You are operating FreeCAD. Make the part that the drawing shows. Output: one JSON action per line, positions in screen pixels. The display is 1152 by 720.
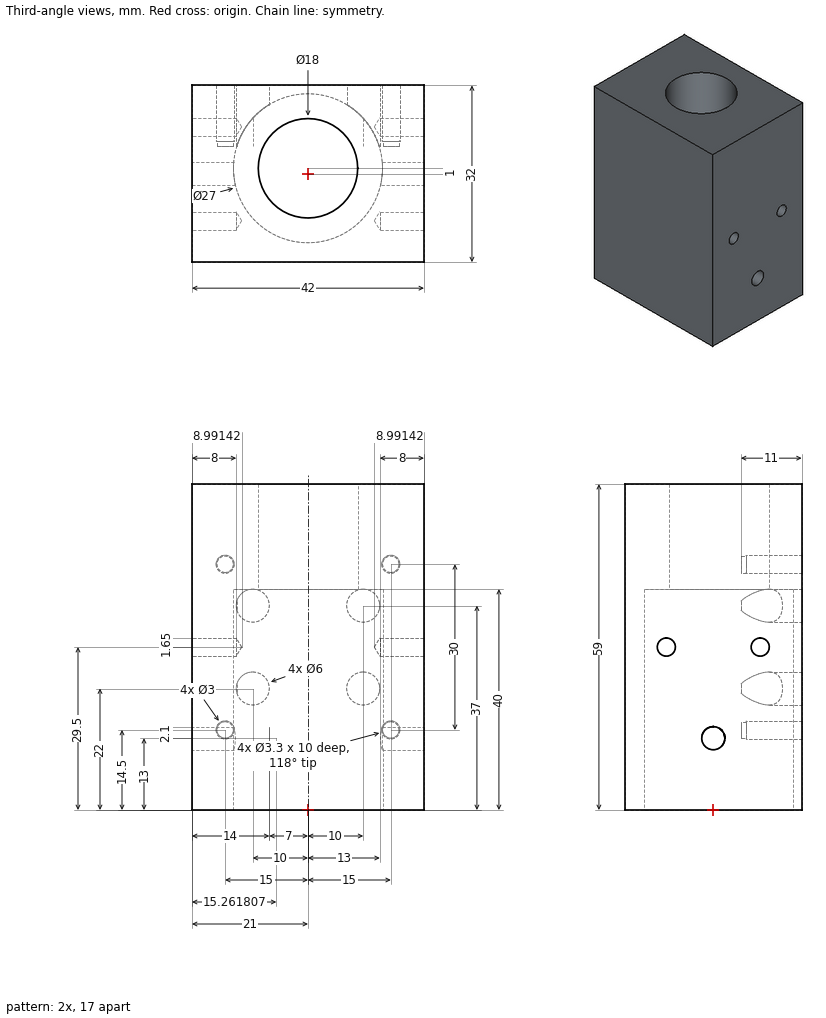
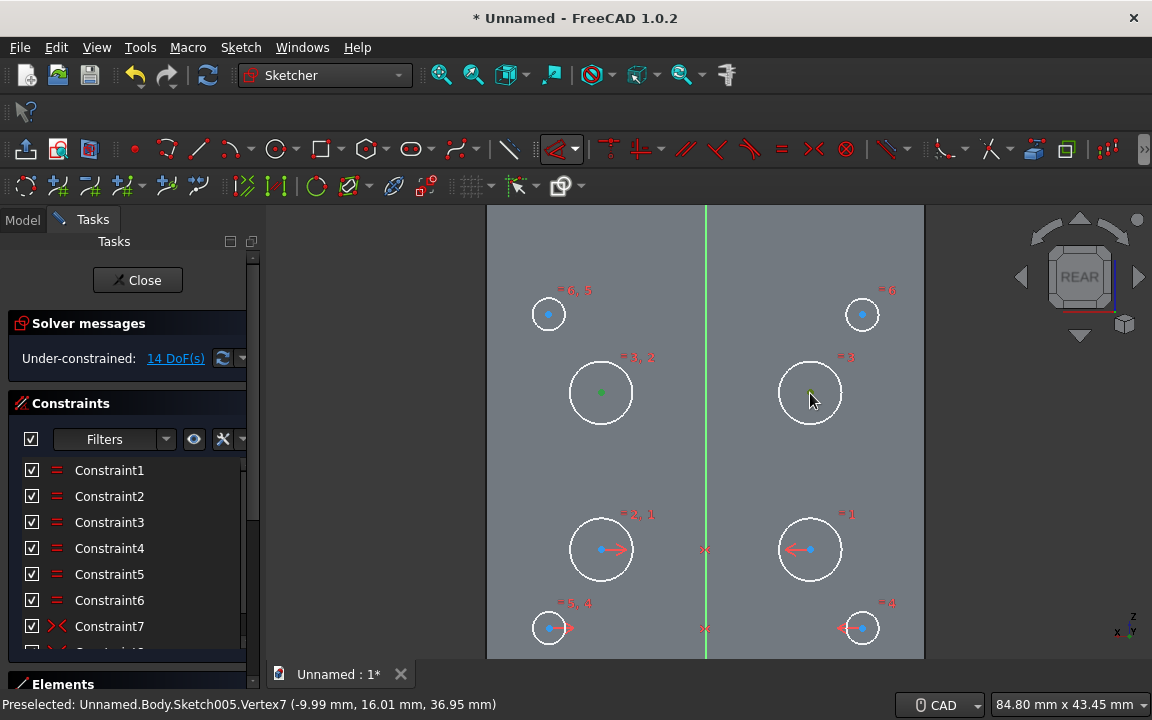
{"action": "left_click", "coordinate": [706, 603]}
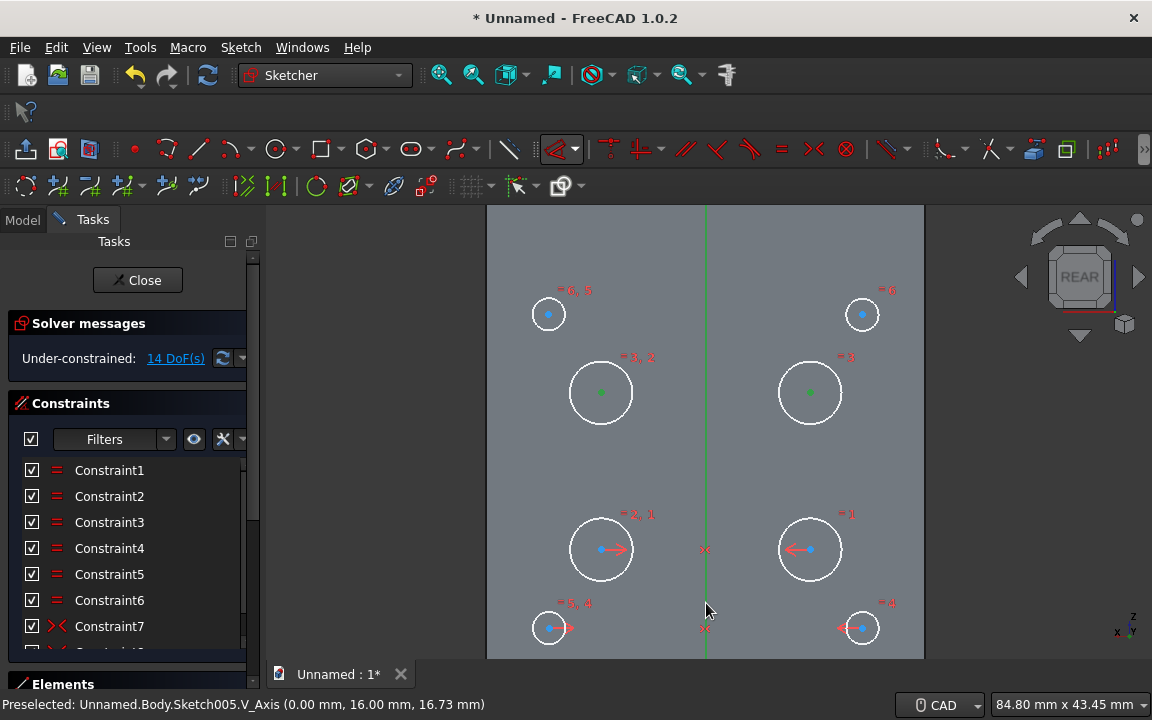
{"action": "left_click", "coordinate": [814, 150]}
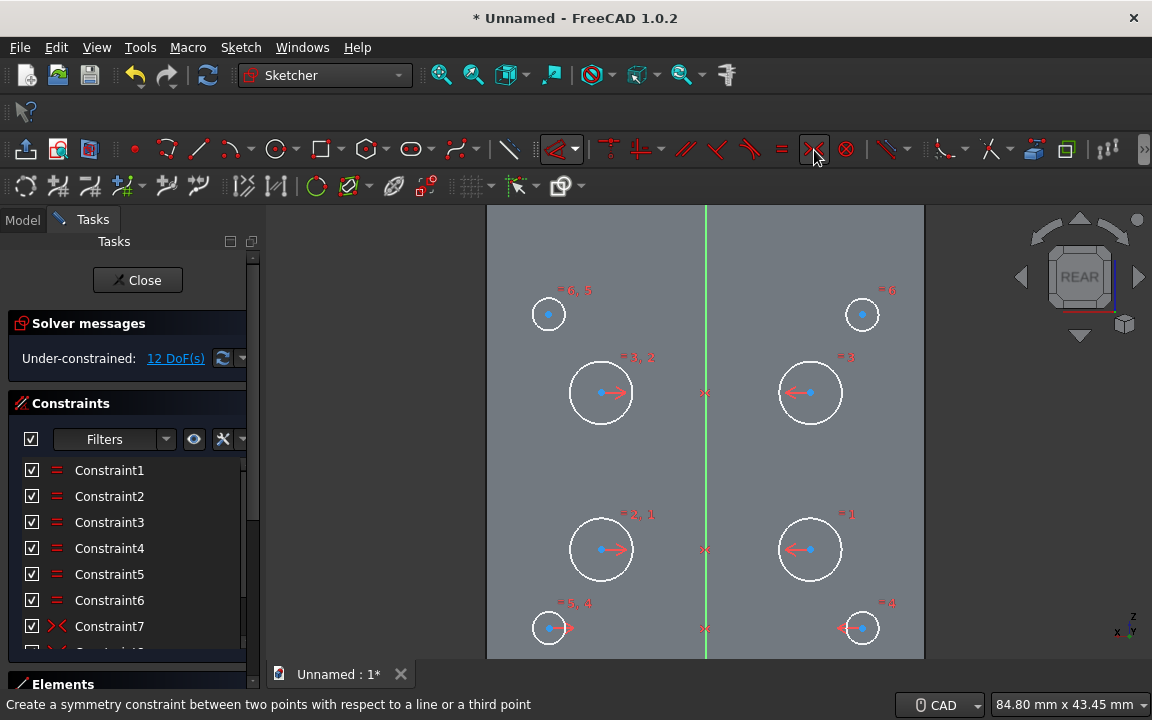
{"action": "left_click", "coordinate": [549, 314]}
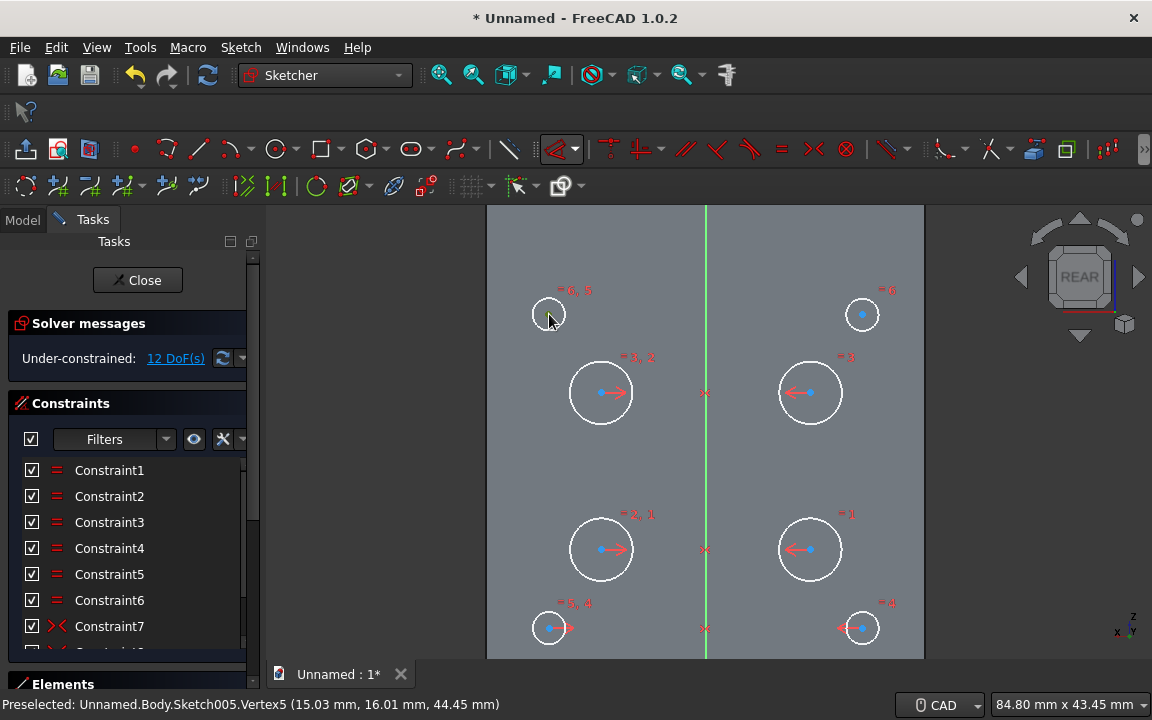
{"action": "left_click", "coordinate": [862, 315]}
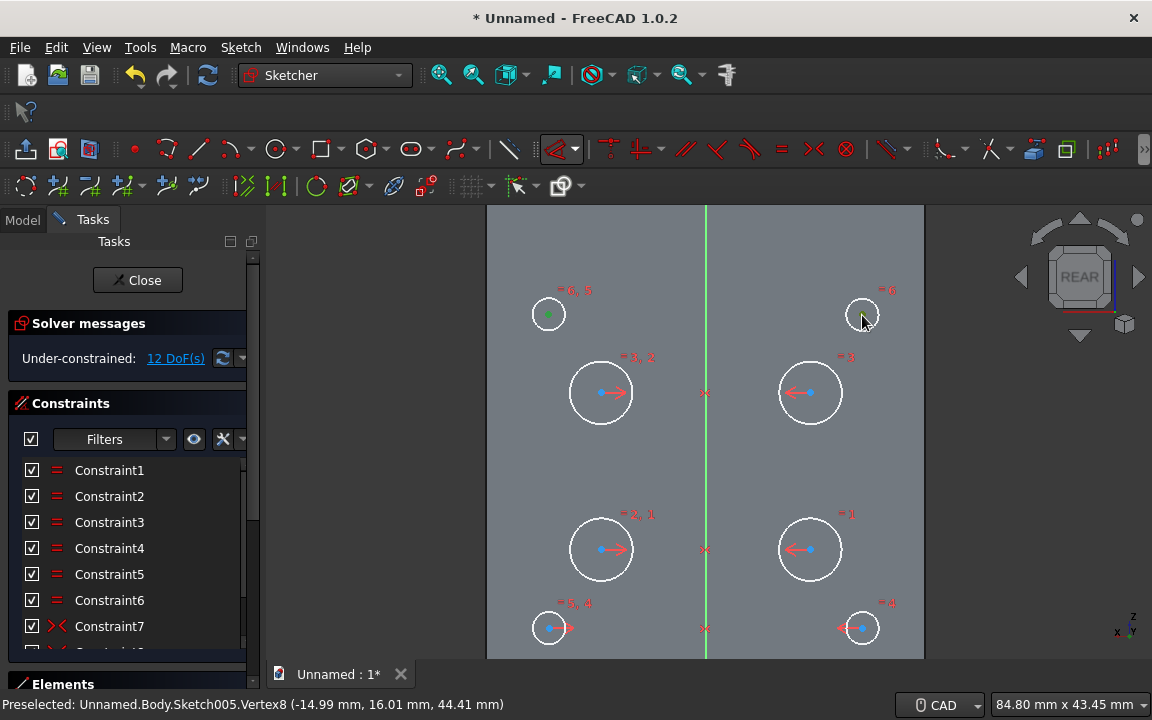
{"action": "left_click", "coordinate": [706, 603]}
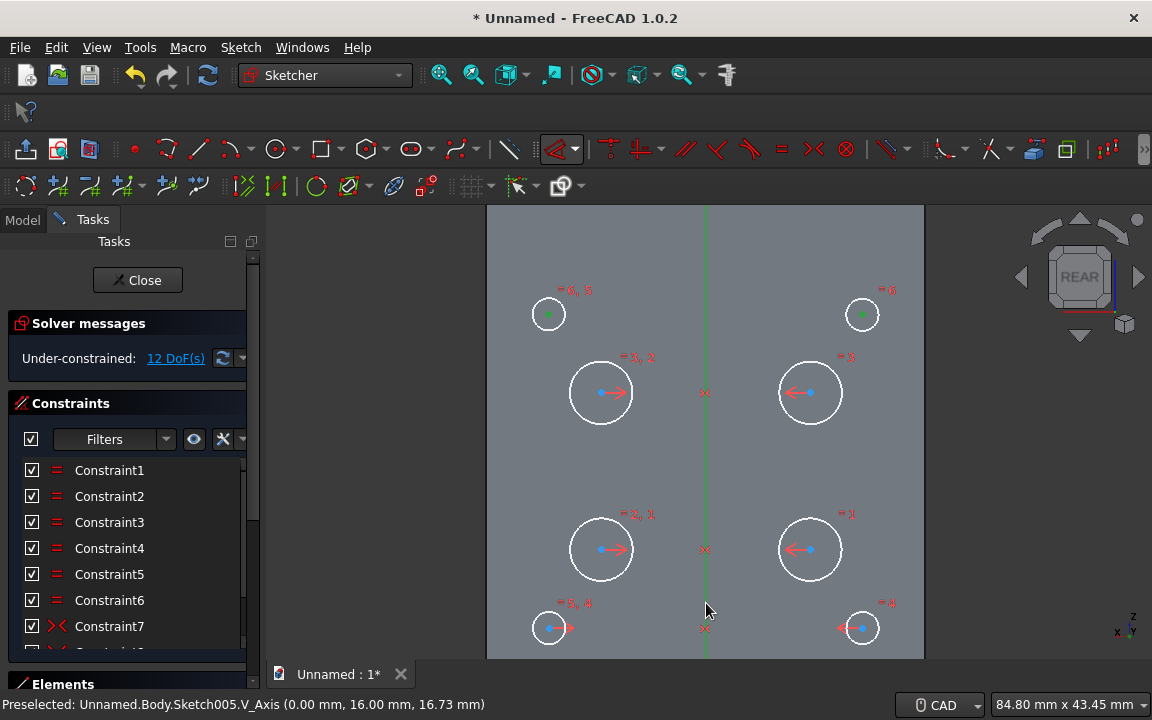
{"action": "key", "text": "s"}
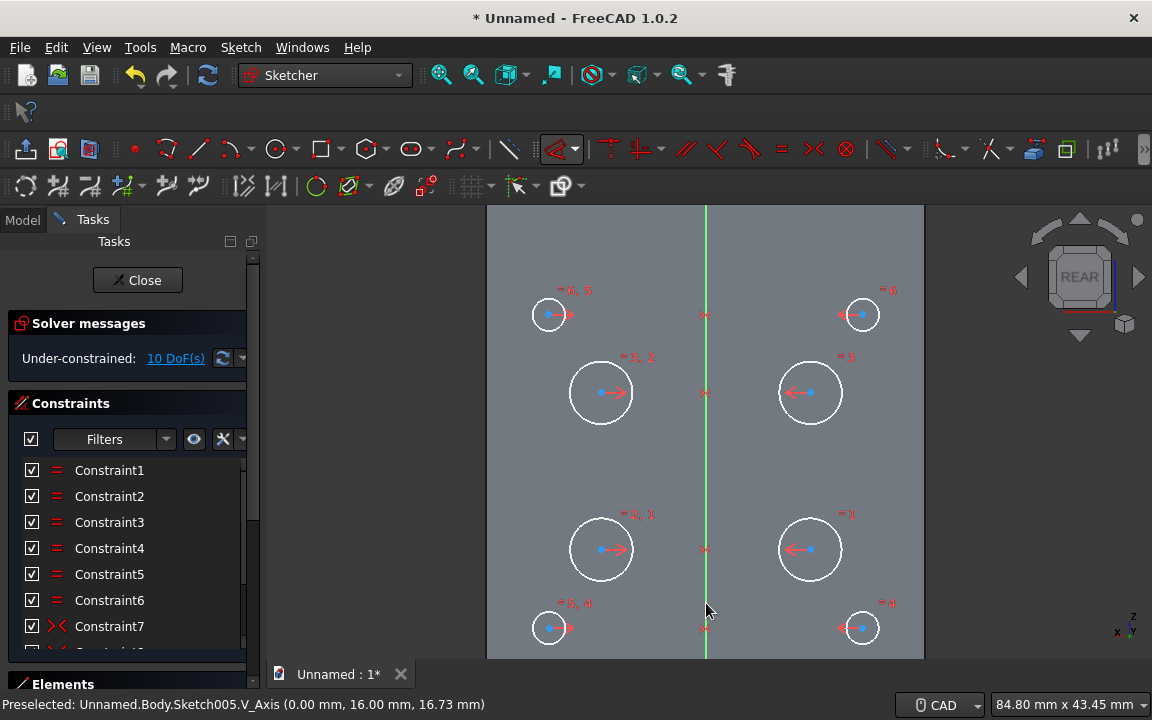
{"action": "scroll", "coordinate": [874, 617], "scroll_direction": "up", "scroll_amount": 2}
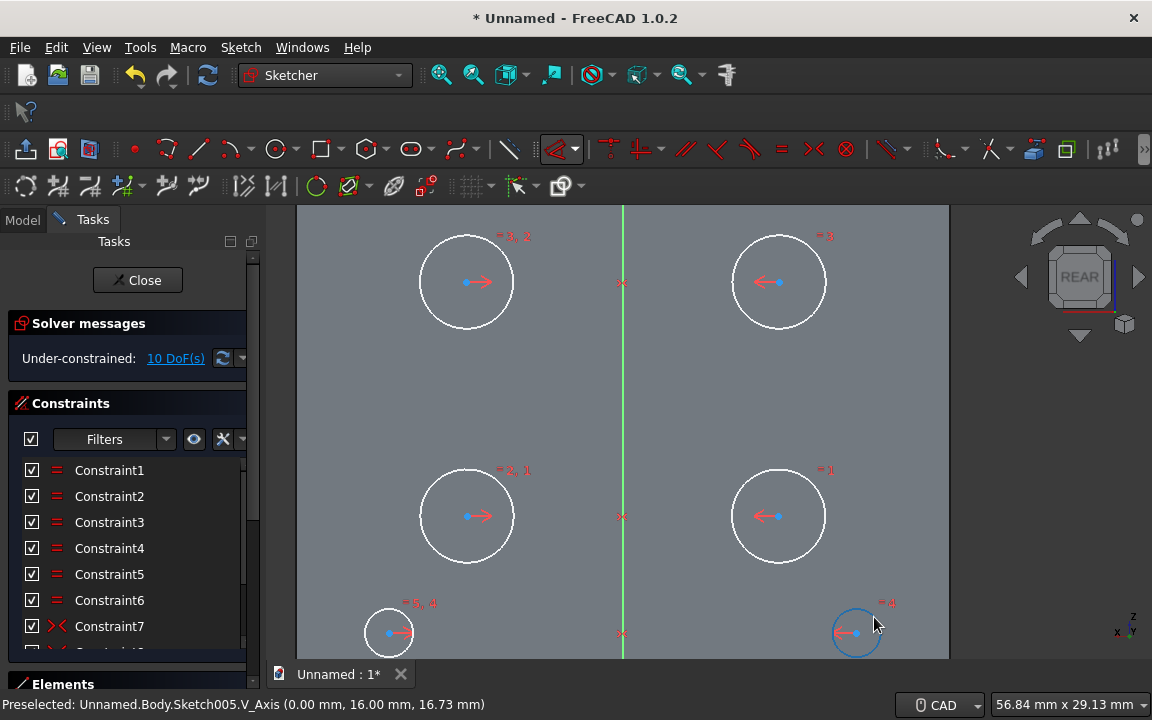
{"action": "left_click", "coordinate": [874, 616]}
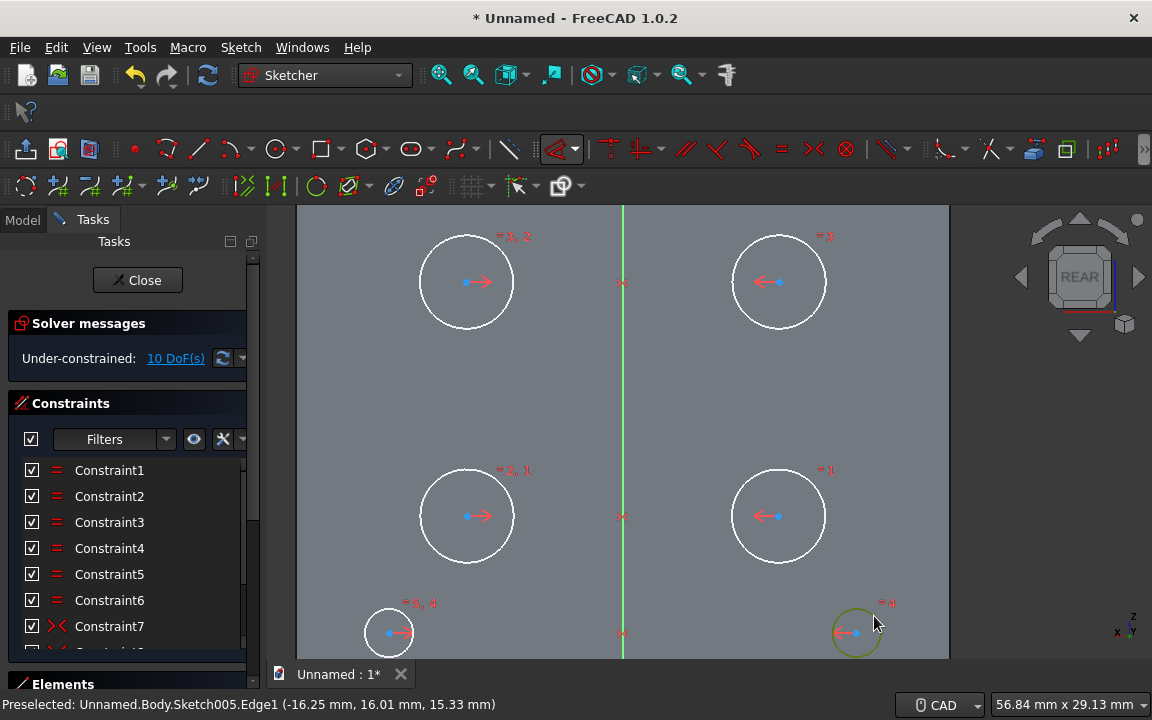
{"action": "key", "text": "k o"}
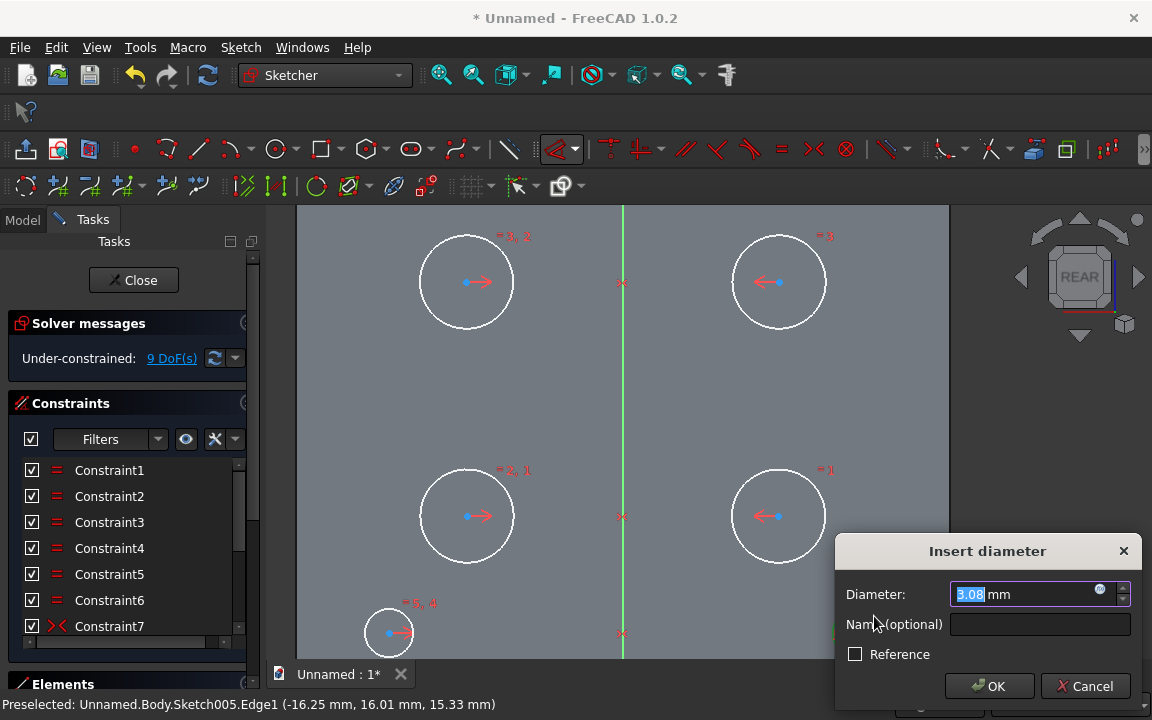
{"action": "type", "text": "3"}
{"action": "key", "text": "Return"}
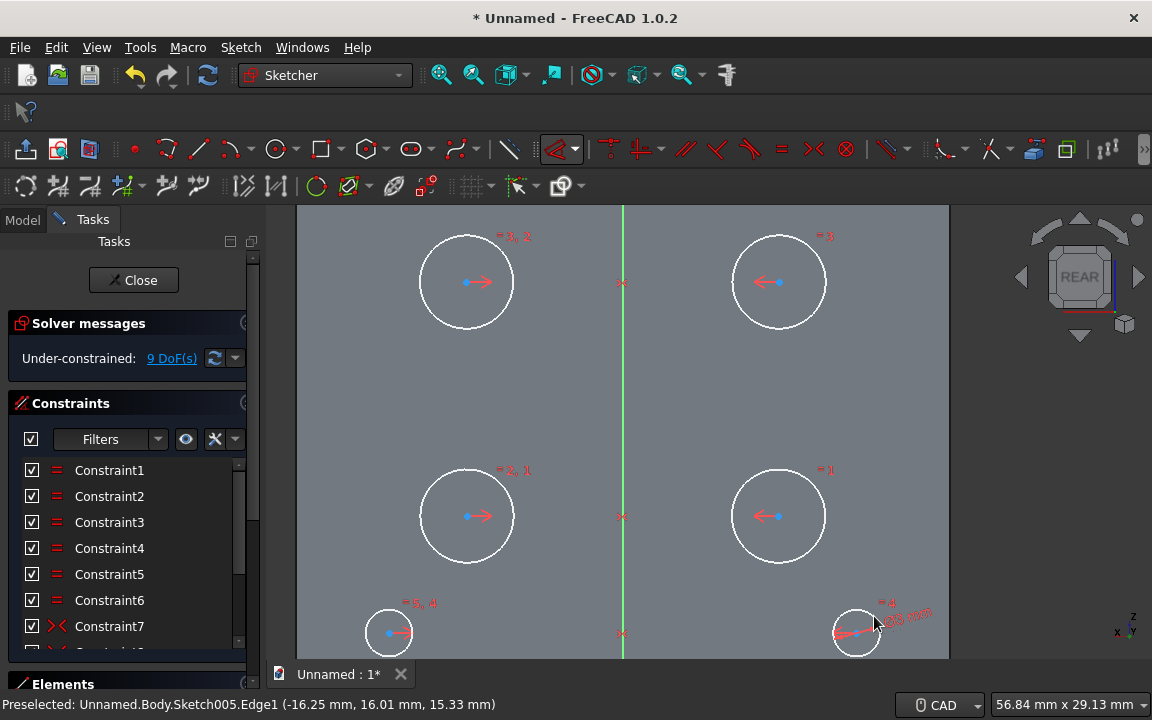
{"action": "left_click", "coordinate": [812, 483]}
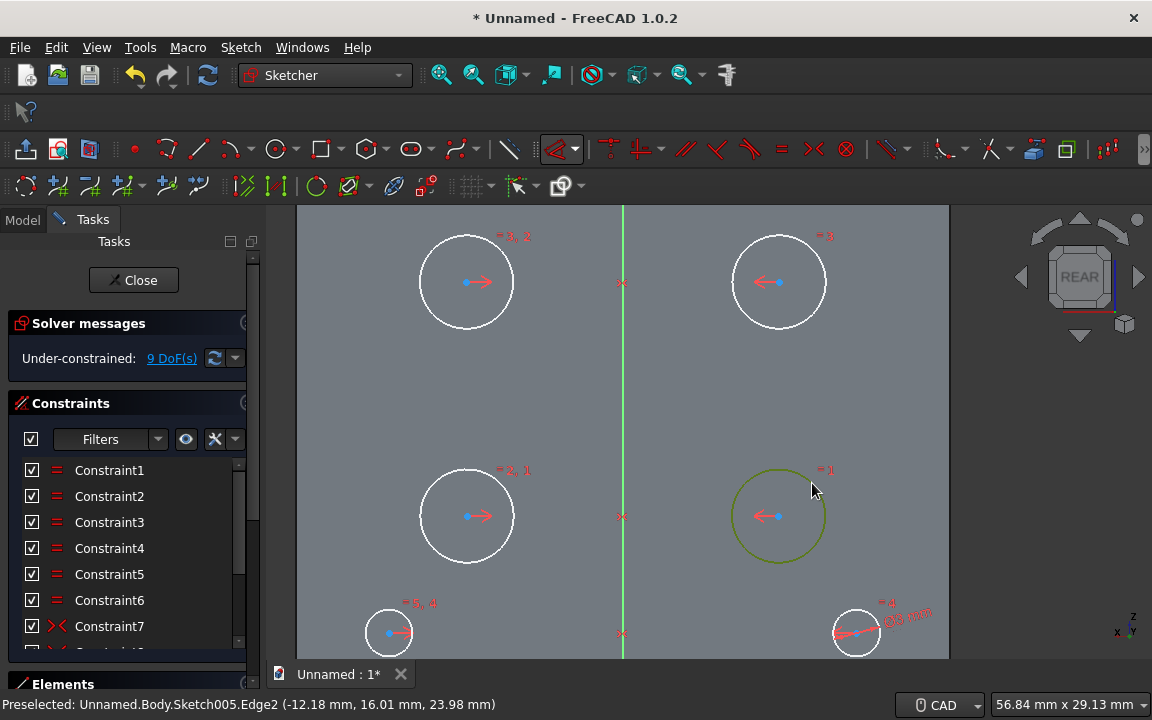
{"action": "key", "text": "k o"}